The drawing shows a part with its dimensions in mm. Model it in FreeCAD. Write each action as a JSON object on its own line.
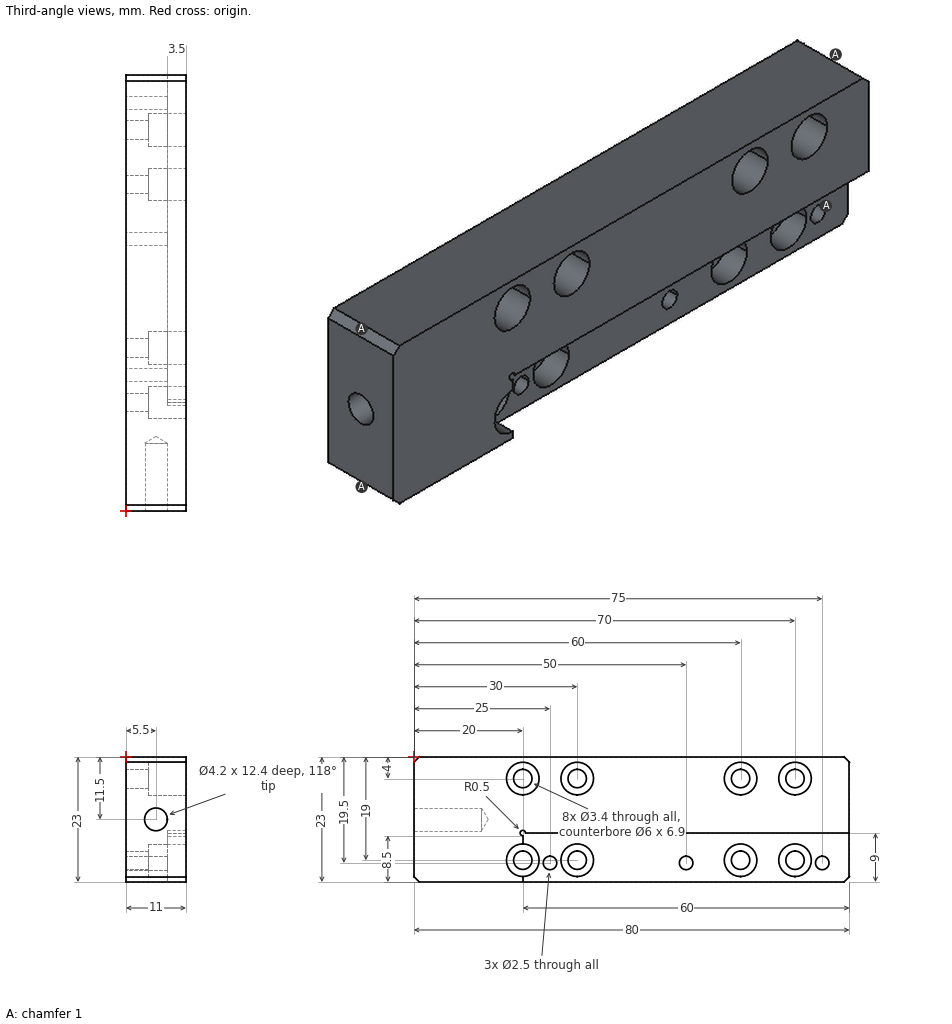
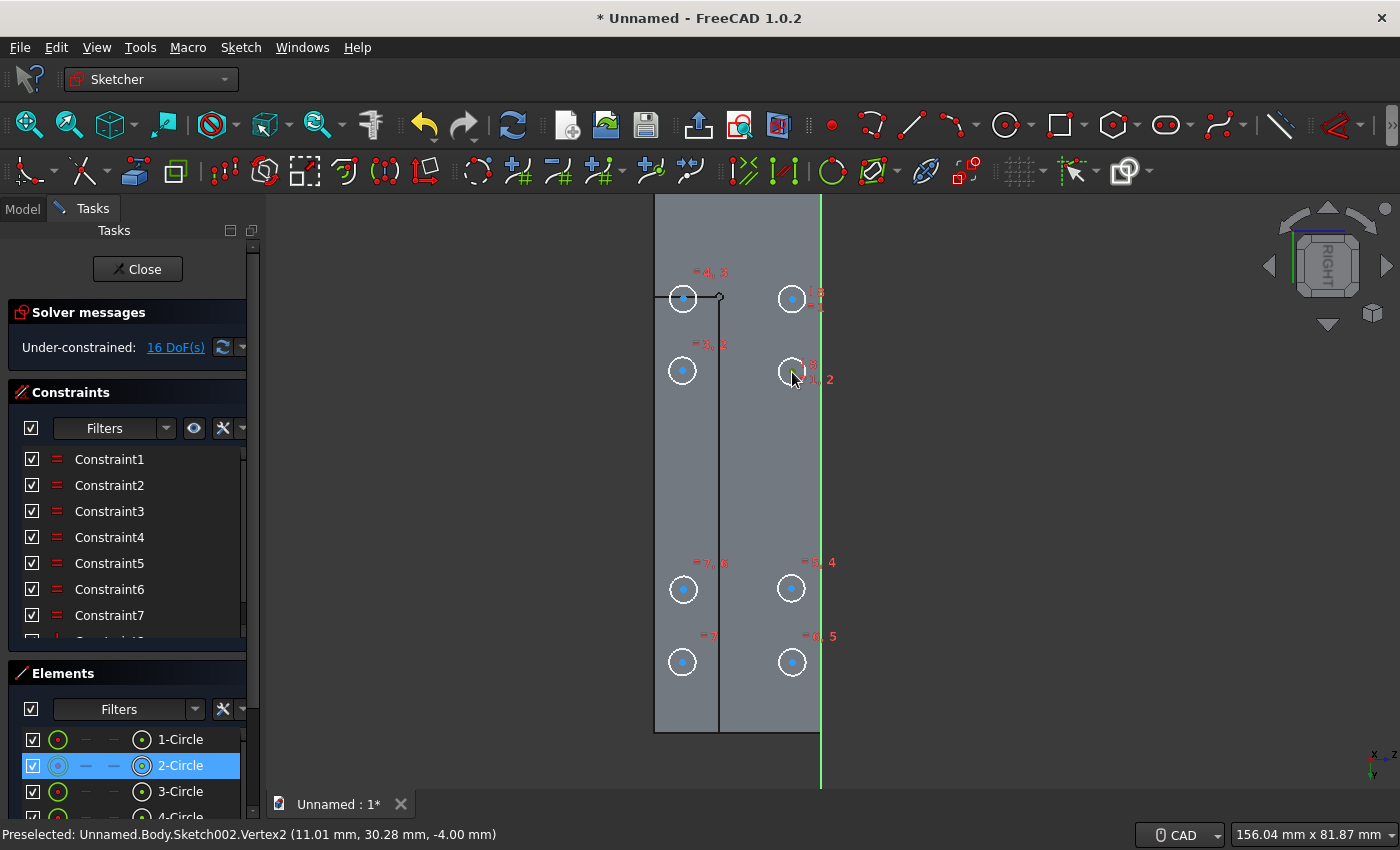
{"action": "left_click", "coordinate": [682, 371]}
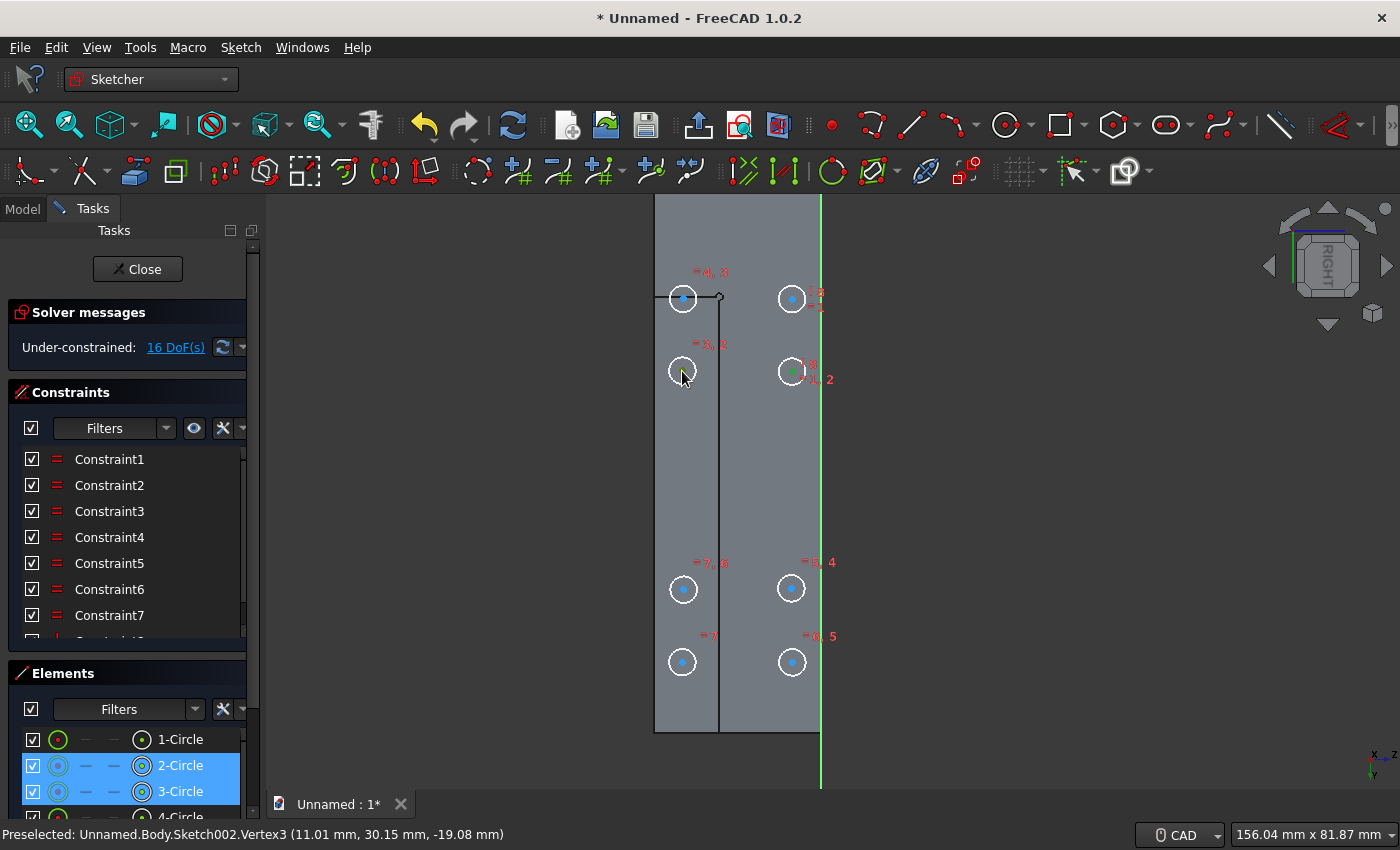
{"action": "key", "text": "h"}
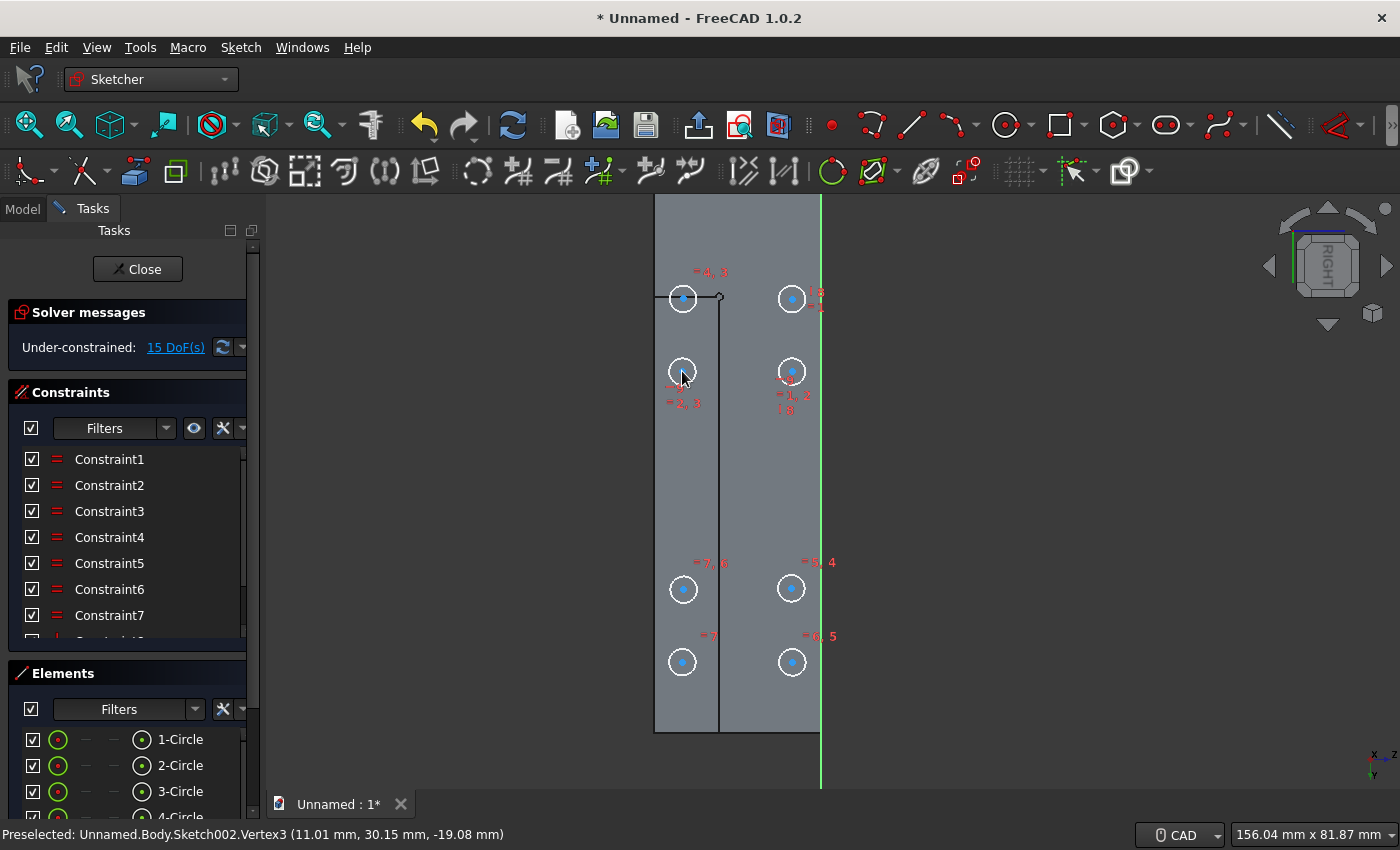
{"action": "left_click", "coordinate": [682, 372]}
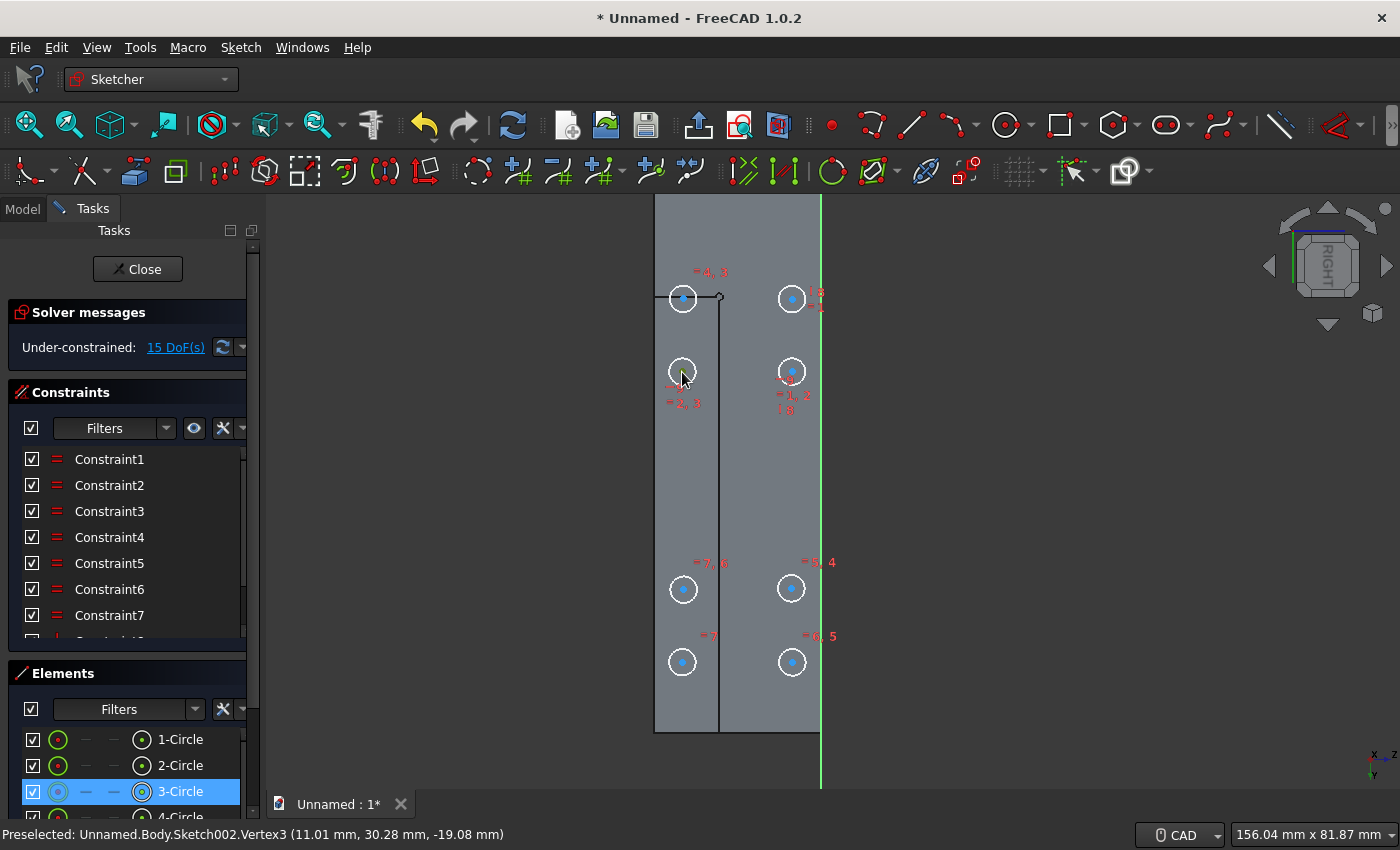
{"action": "left_click", "coordinate": [683, 299]}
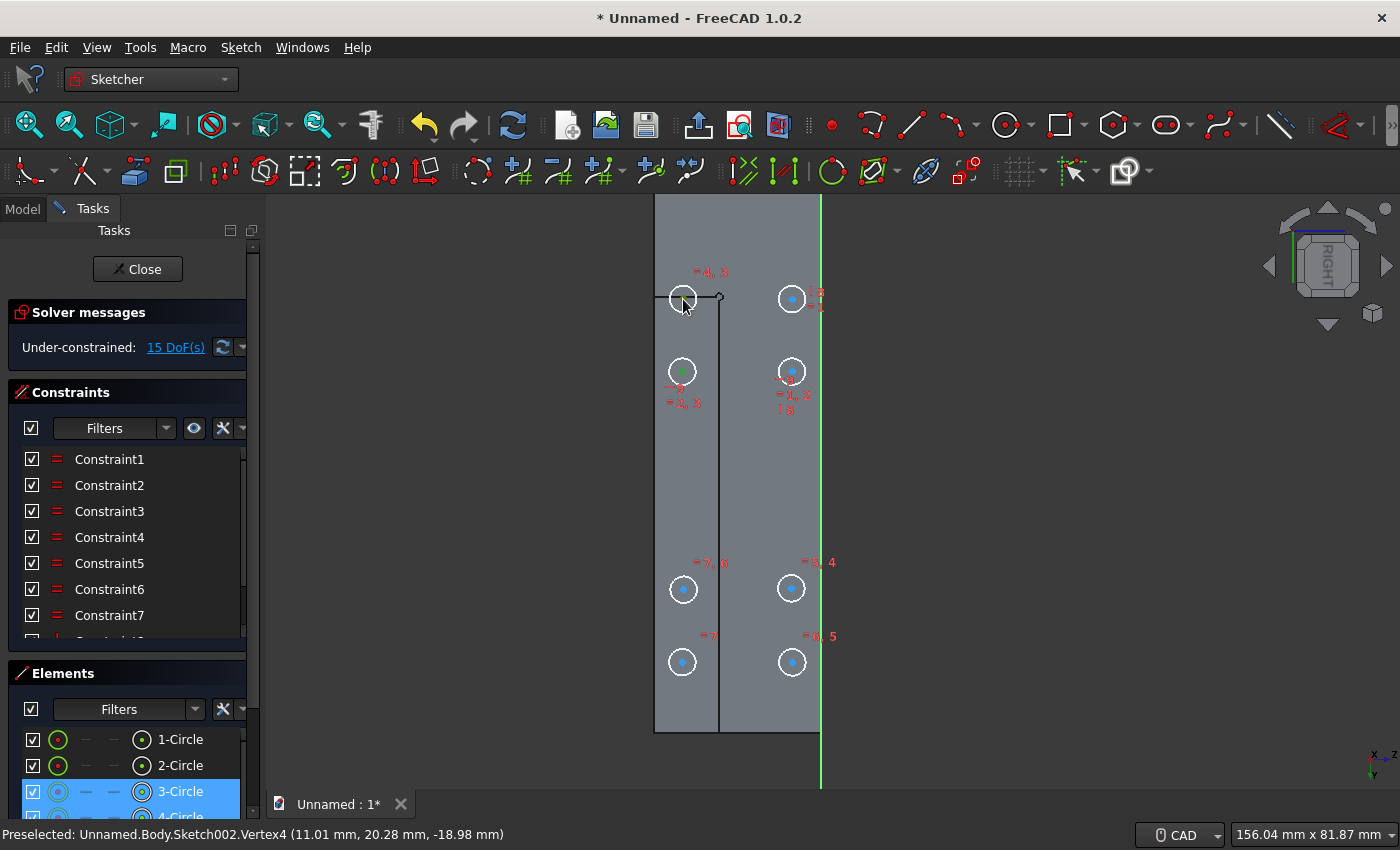
{"action": "key", "text": "v"}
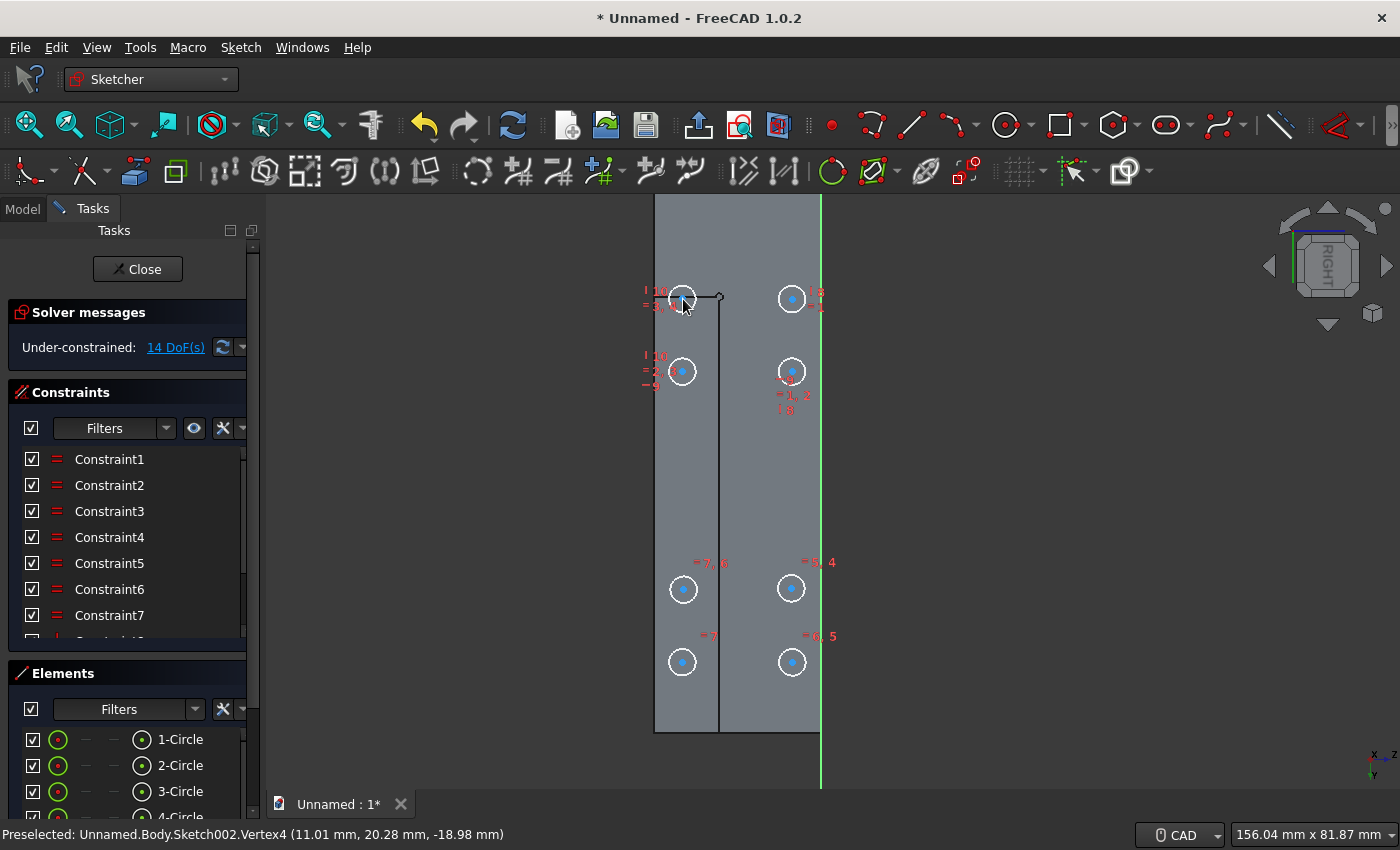
{"action": "left_click", "coordinate": [792, 299]}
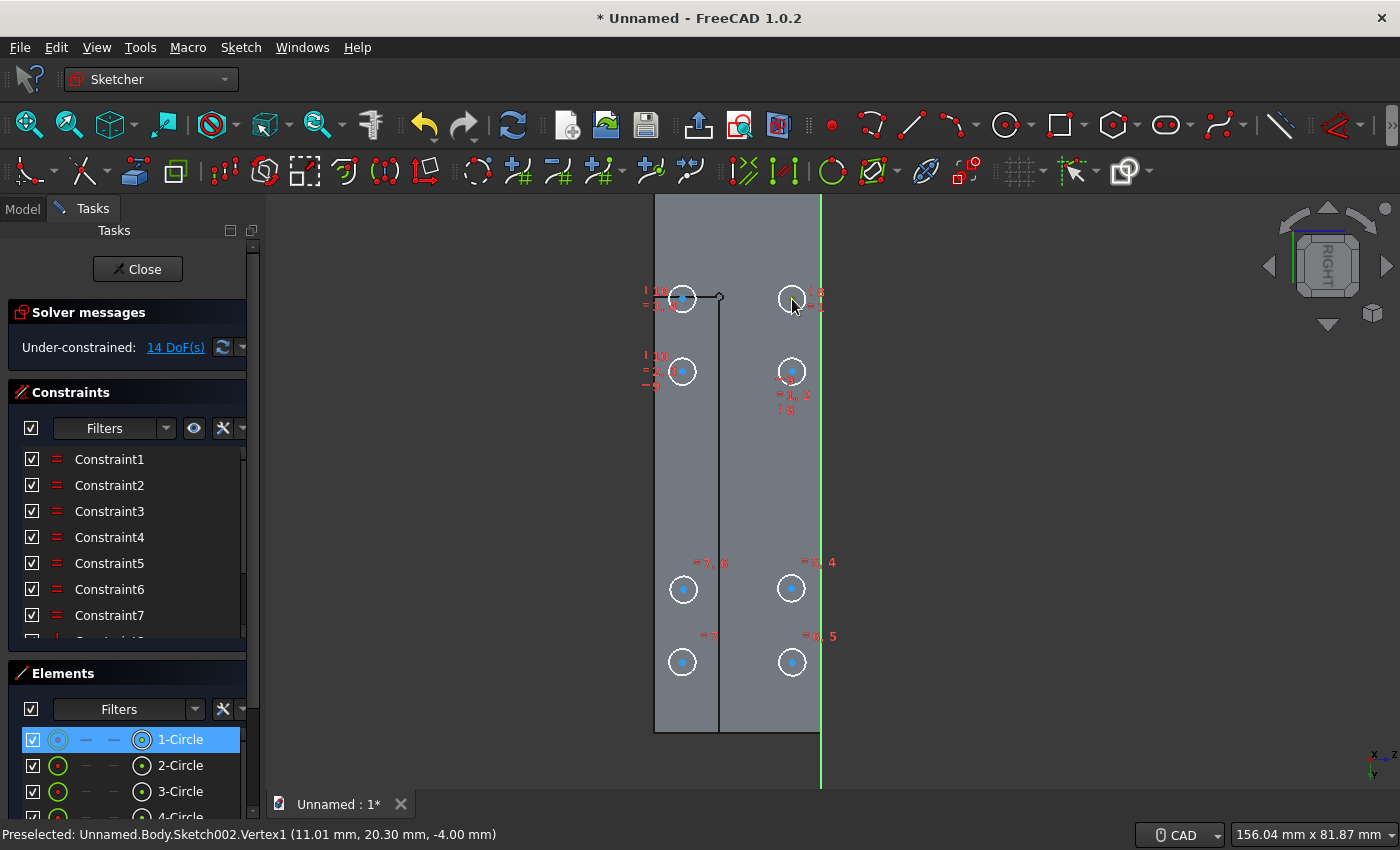
{"action": "left_click", "coordinate": [682, 299]}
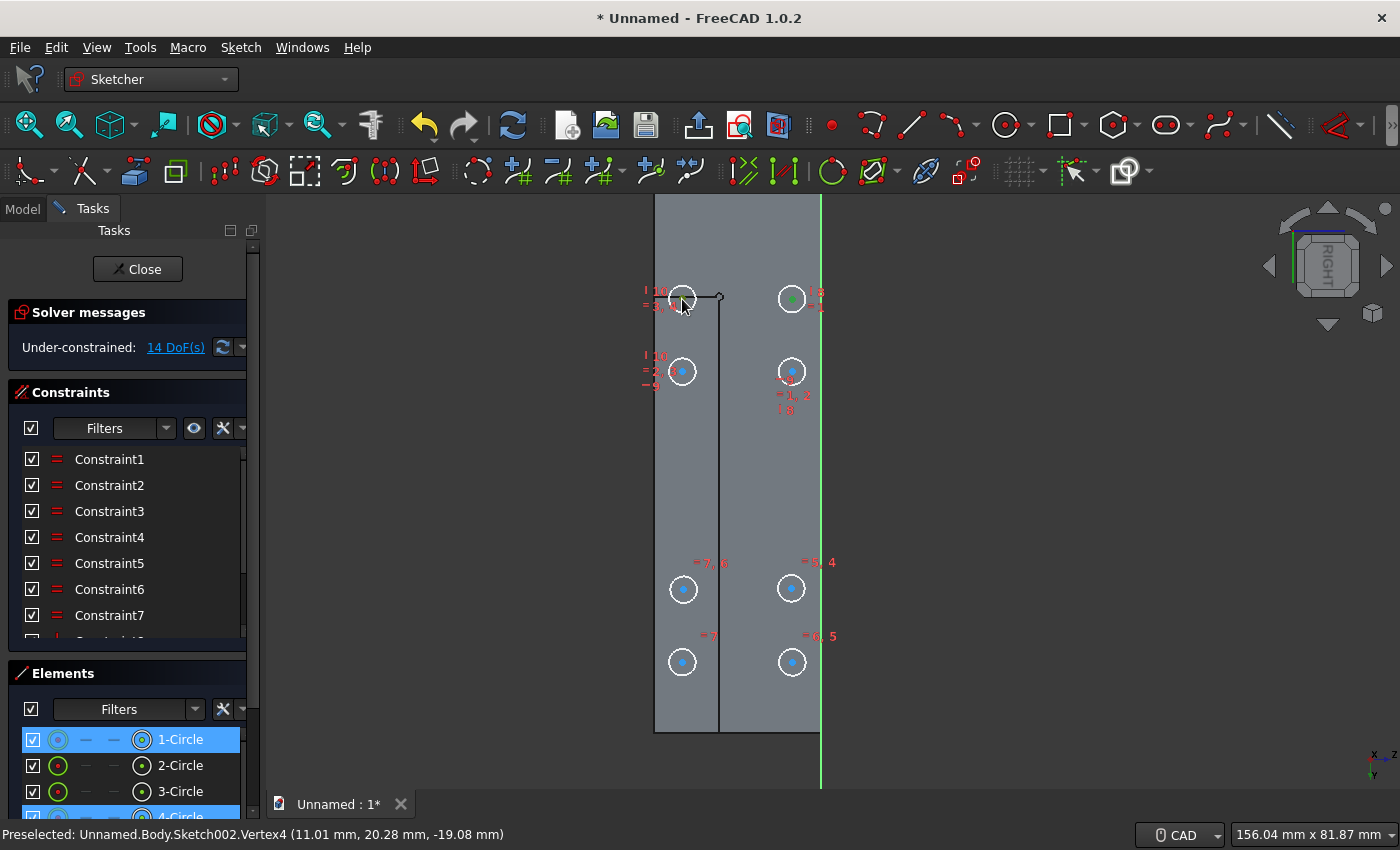
{"action": "key", "text": "h"}